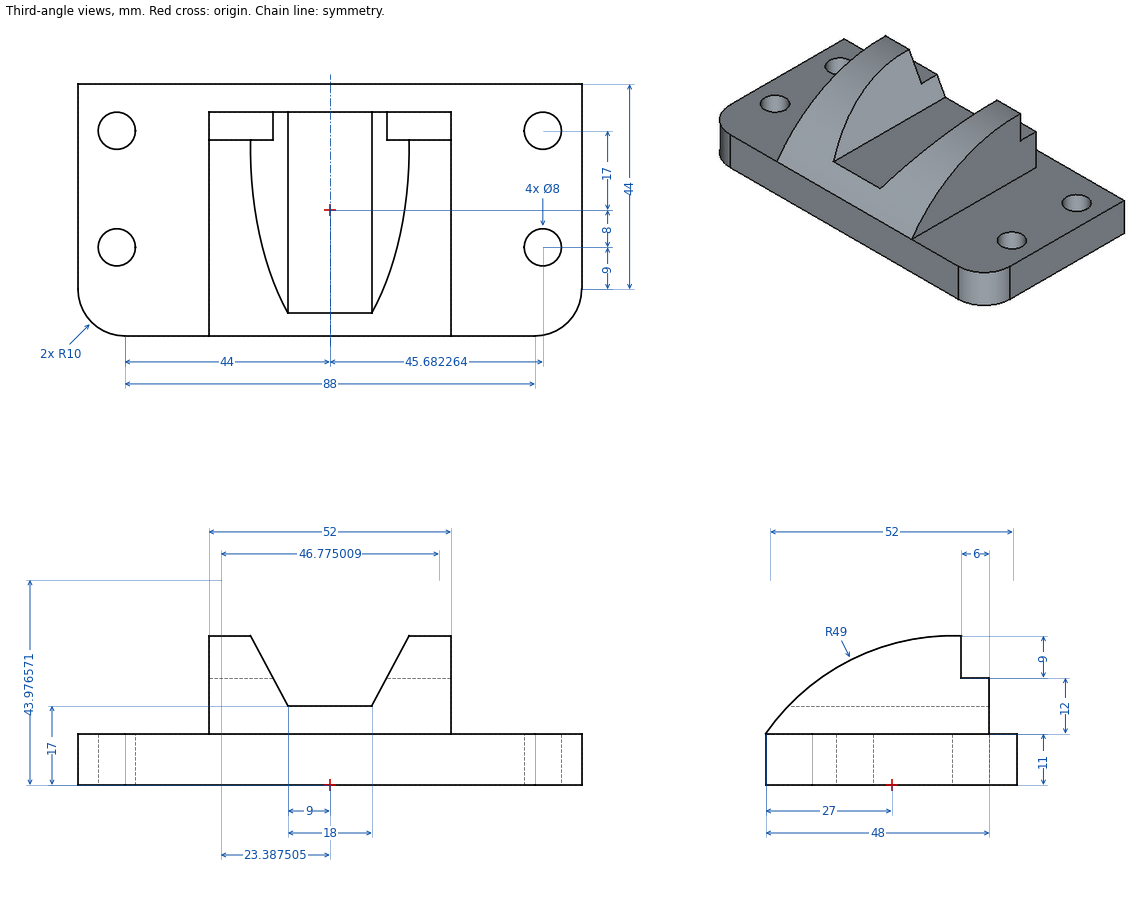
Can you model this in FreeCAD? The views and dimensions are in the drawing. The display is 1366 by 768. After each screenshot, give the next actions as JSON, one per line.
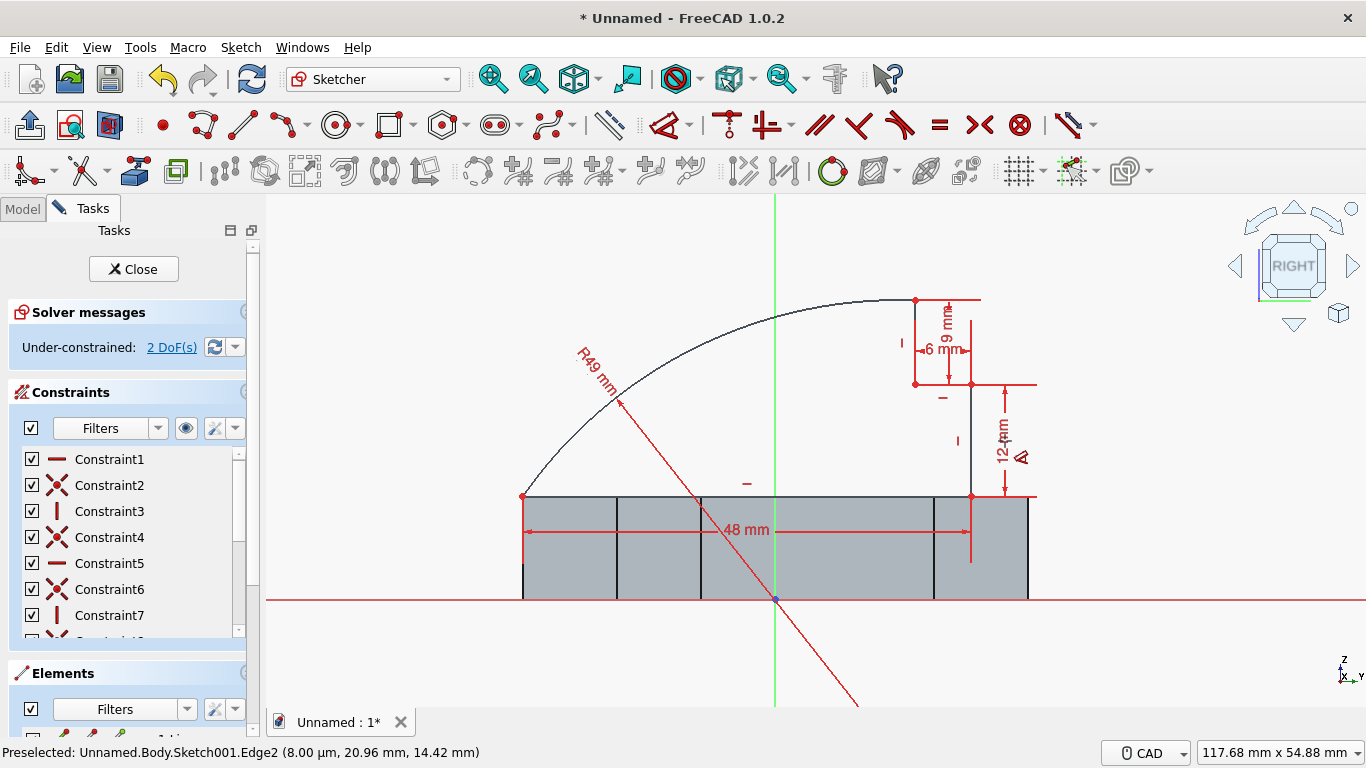
{"action": "left_click", "coordinate": [523, 497]}
{"action": "left_click", "coordinate": [649, 634]}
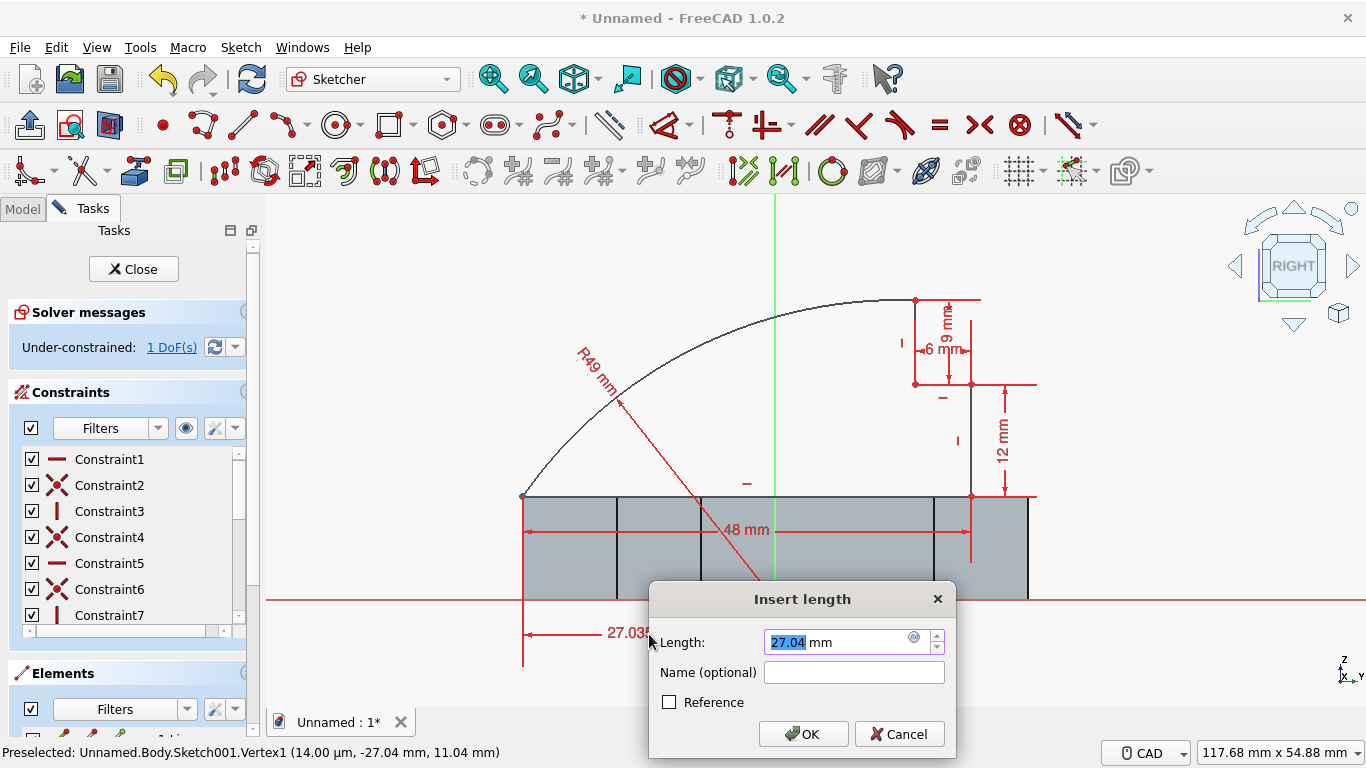
{"action": "type", "text": "27"}
{"action": "key", "text": "Return"}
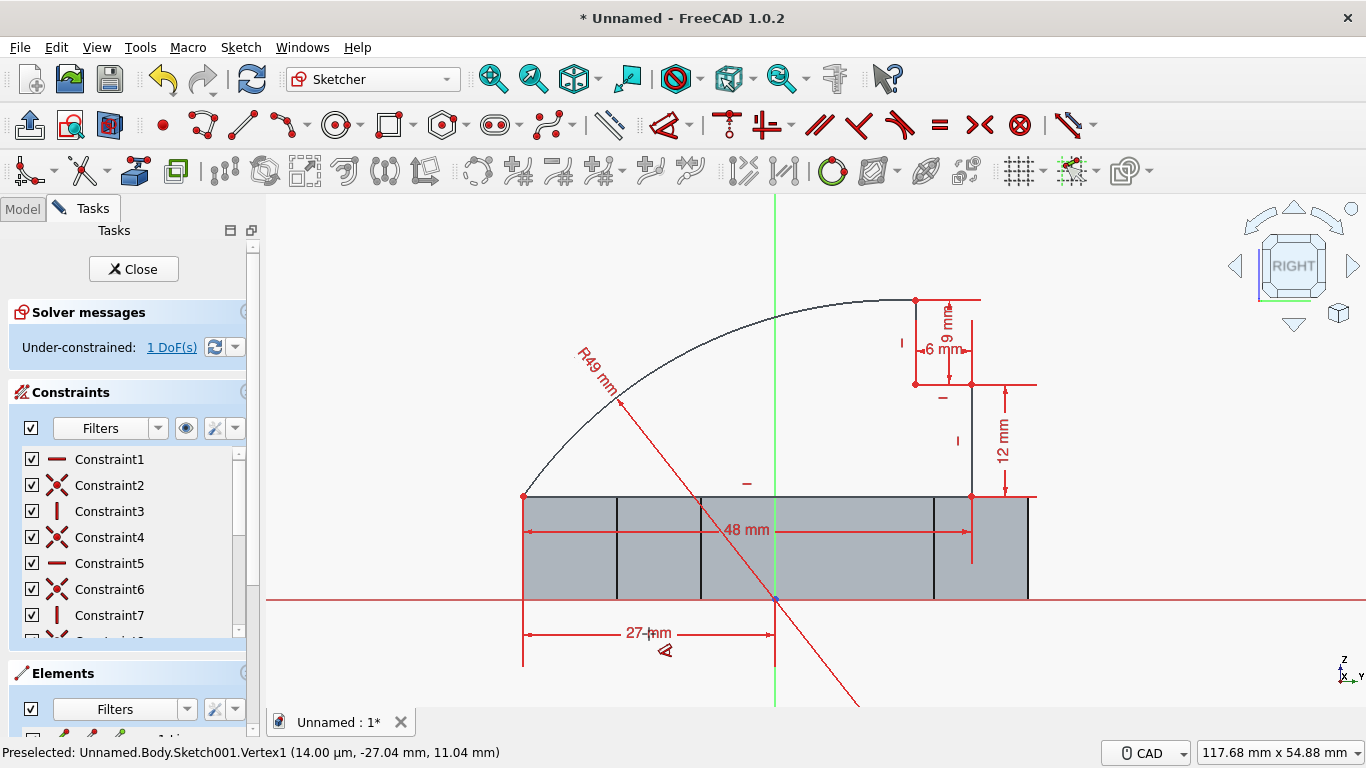
{"action": "left_click", "coordinate": [523, 497]}
{"action": "left_click", "coordinate": [489, 548]}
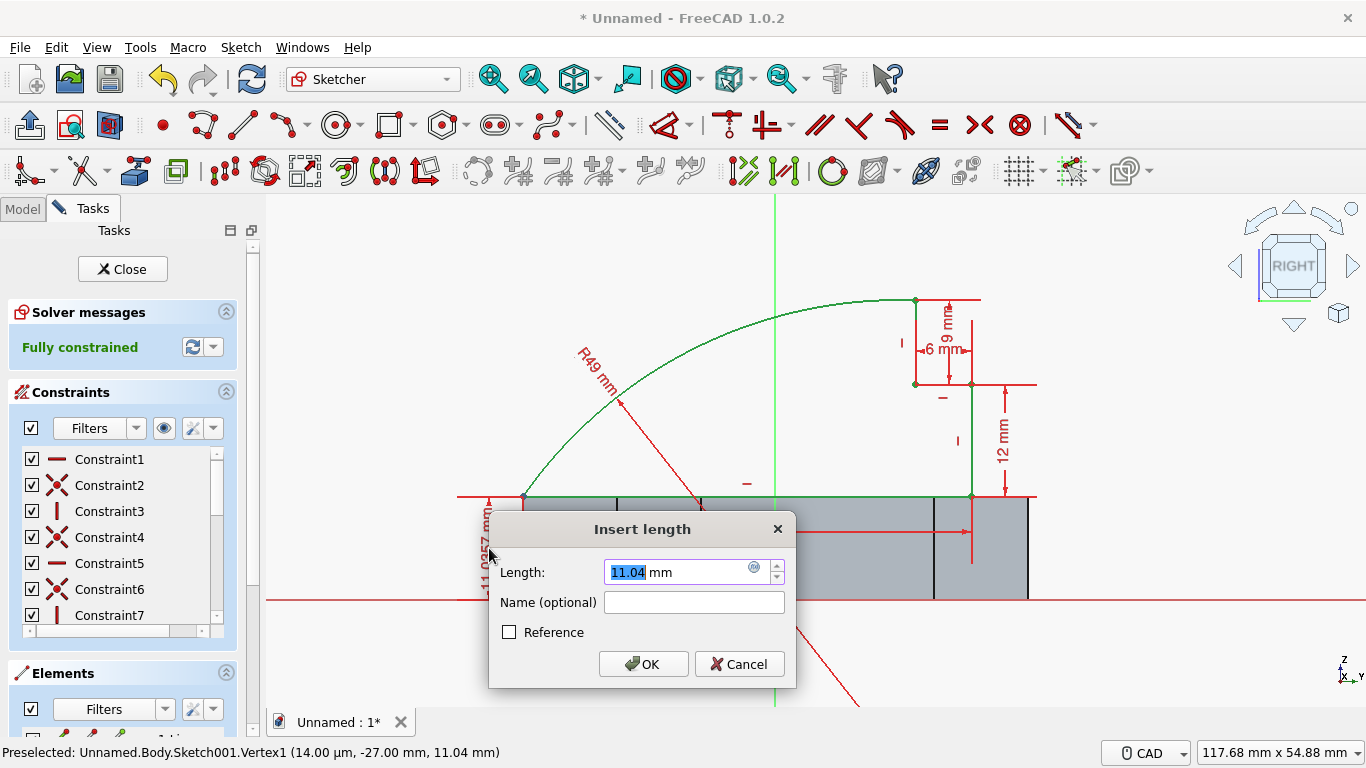
{"action": "type", "text": "11"}
{"action": "key", "text": "Return"}
{"action": "key", "text": "Escape"}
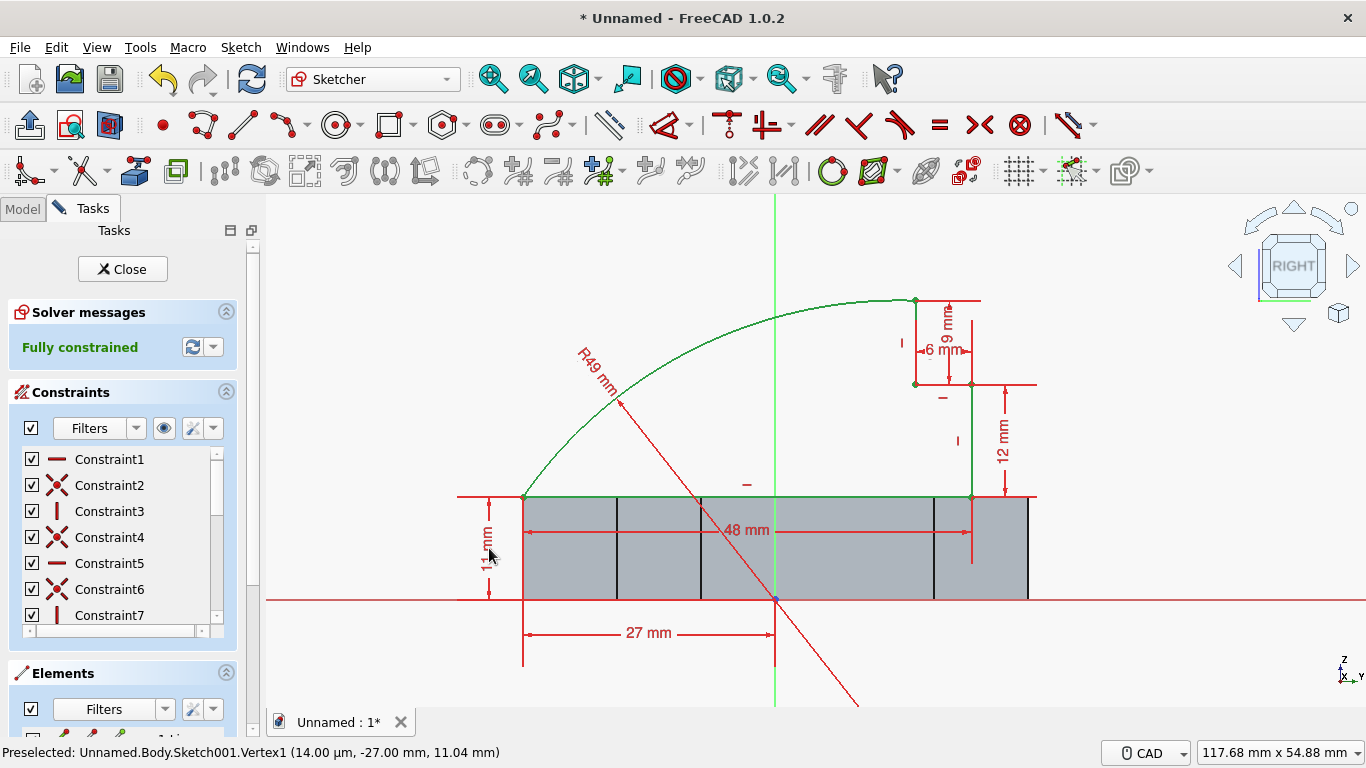
{"action": "left_click", "coordinate": [123, 269]}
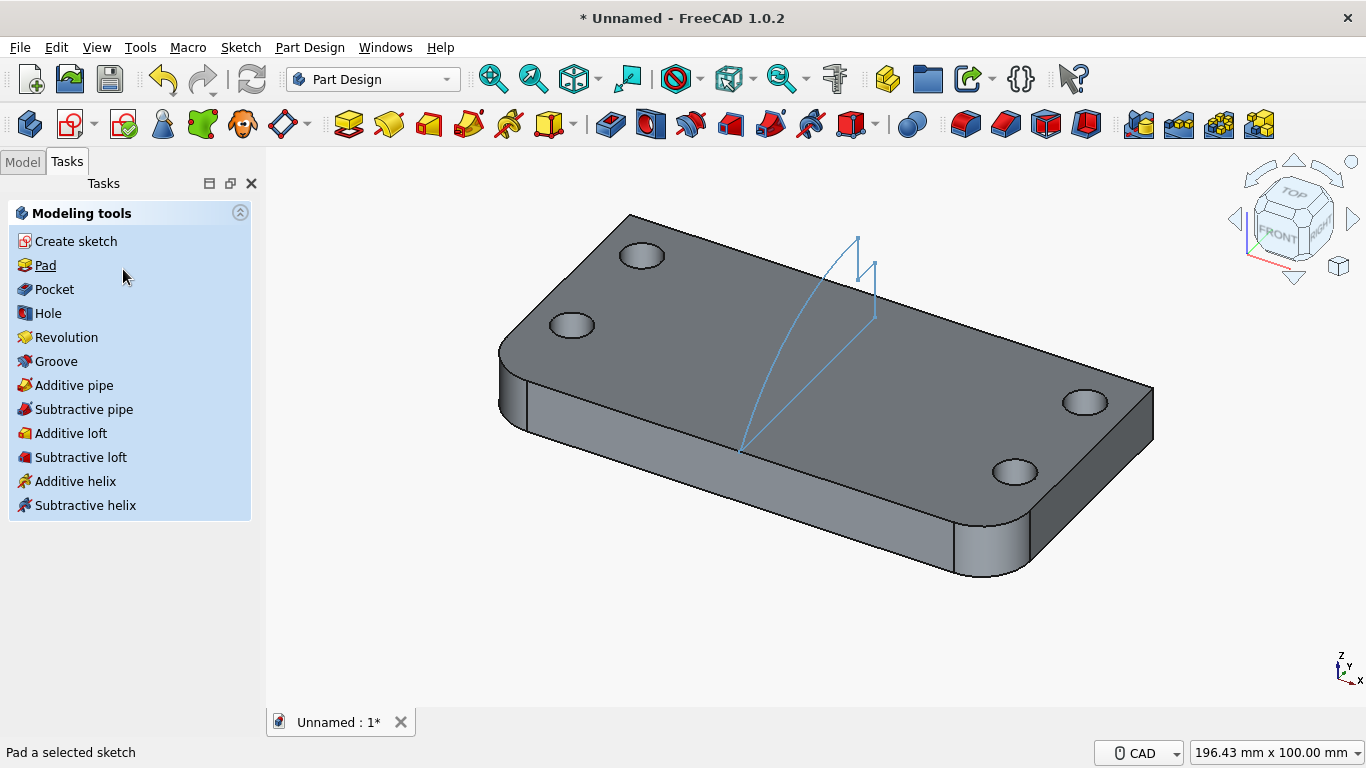
{"action": "left_click", "coordinate": [350, 124]}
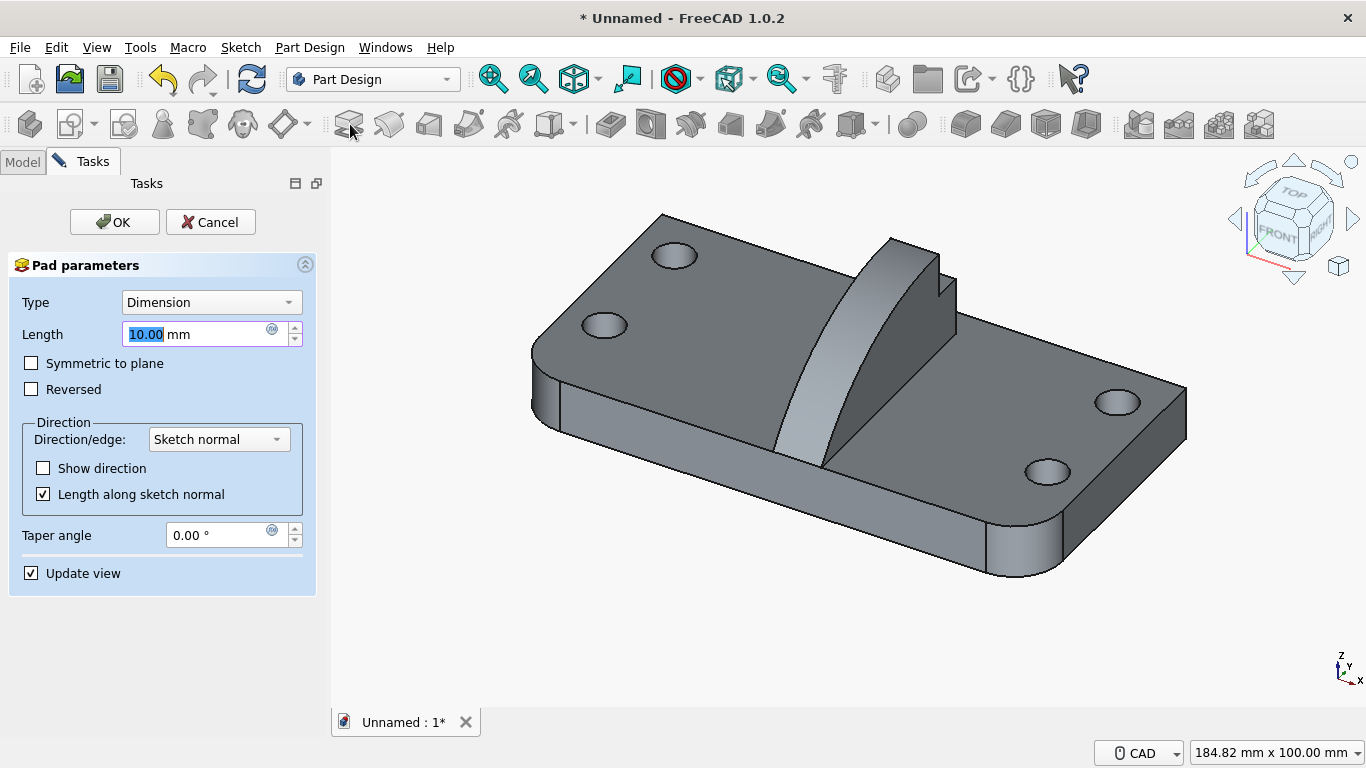
{"action": "type", "text": "52"}
{"action": "key", "text": "Tab"}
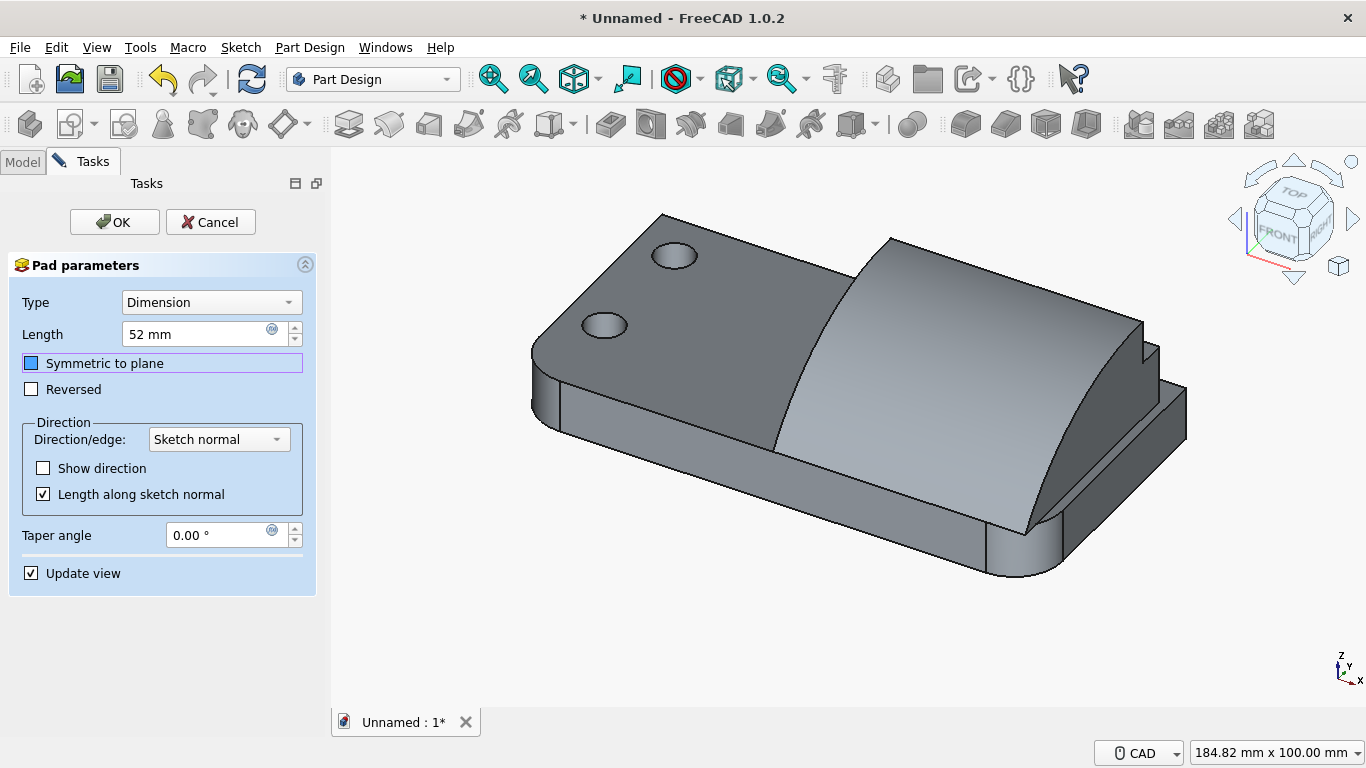
{"action": "left_click", "coordinate": [30, 363]}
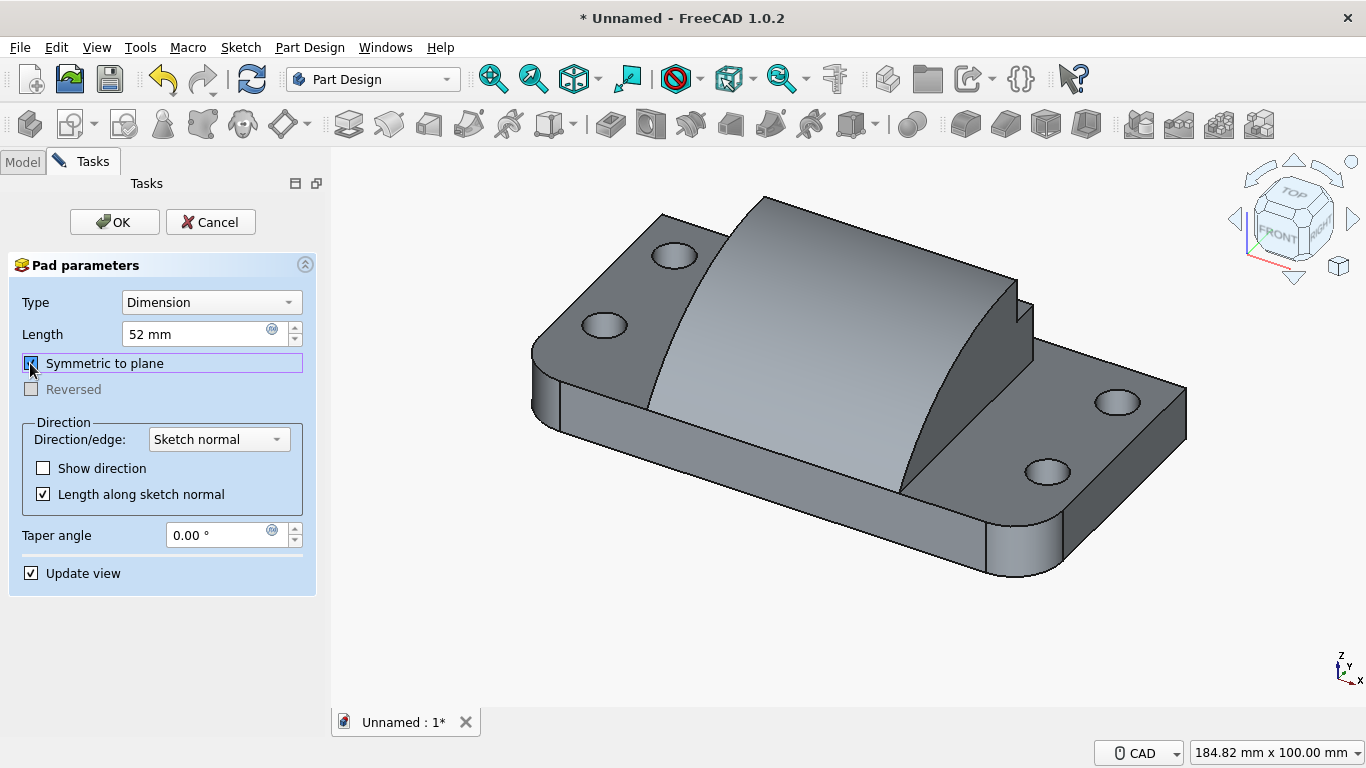
{"action": "left_click", "coordinate": [115, 222]}